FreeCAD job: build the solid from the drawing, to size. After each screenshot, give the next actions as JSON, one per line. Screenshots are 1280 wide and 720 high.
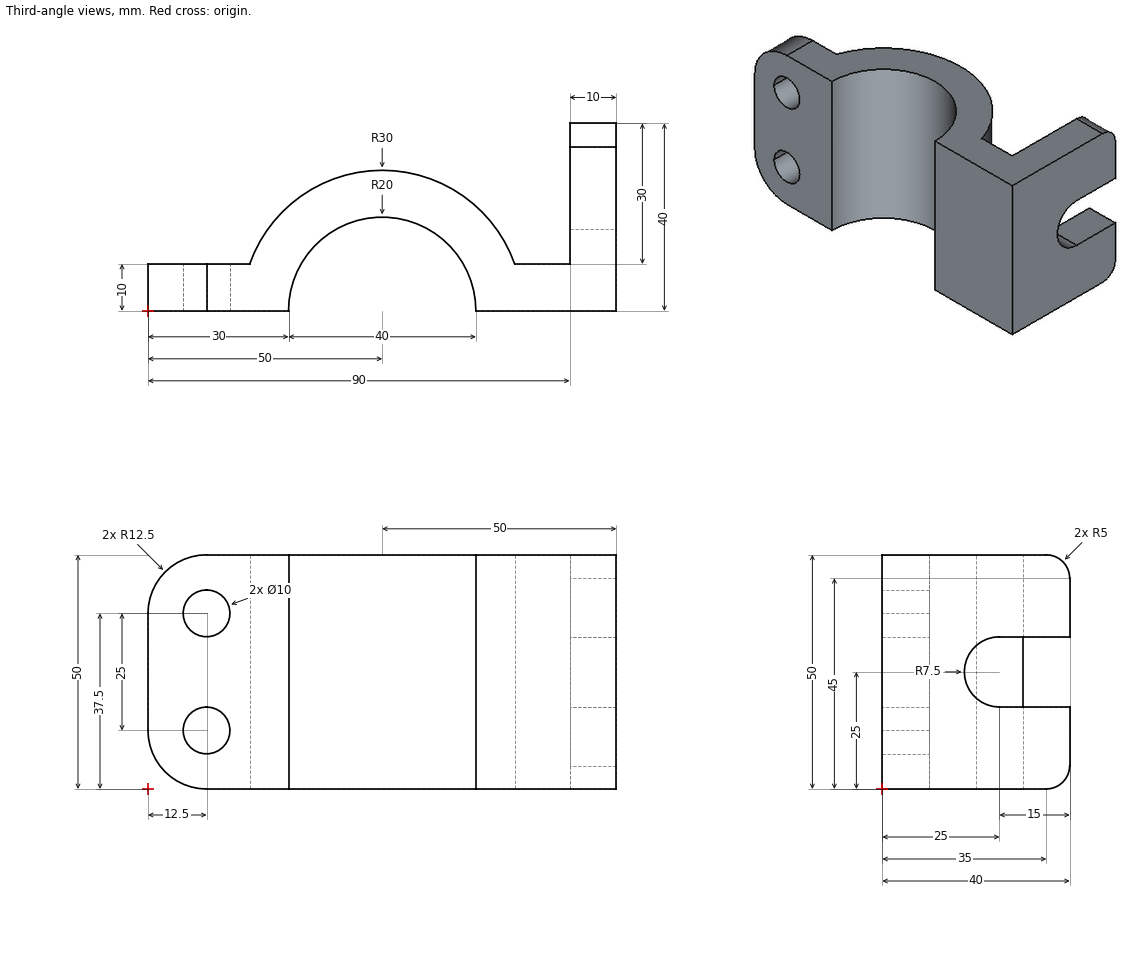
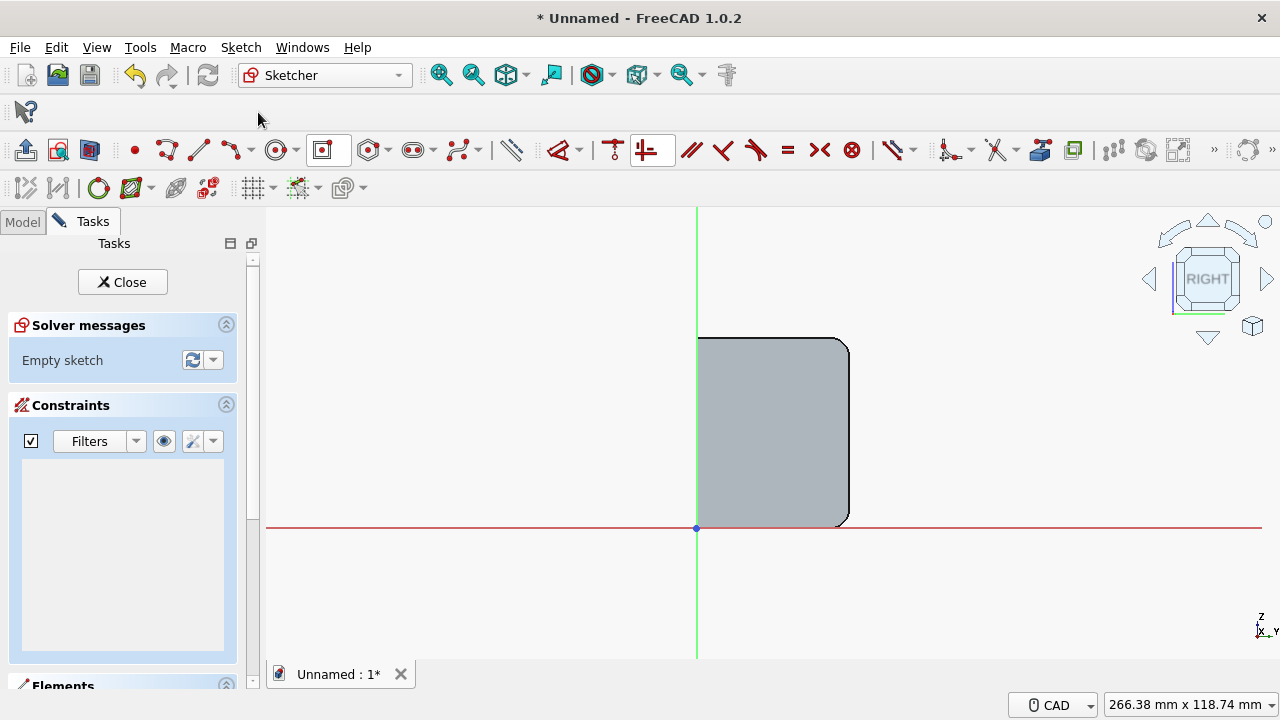
{"action": "scroll", "coordinate": [829, 493], "scroll_direction": "up", "scroll_amount": 4}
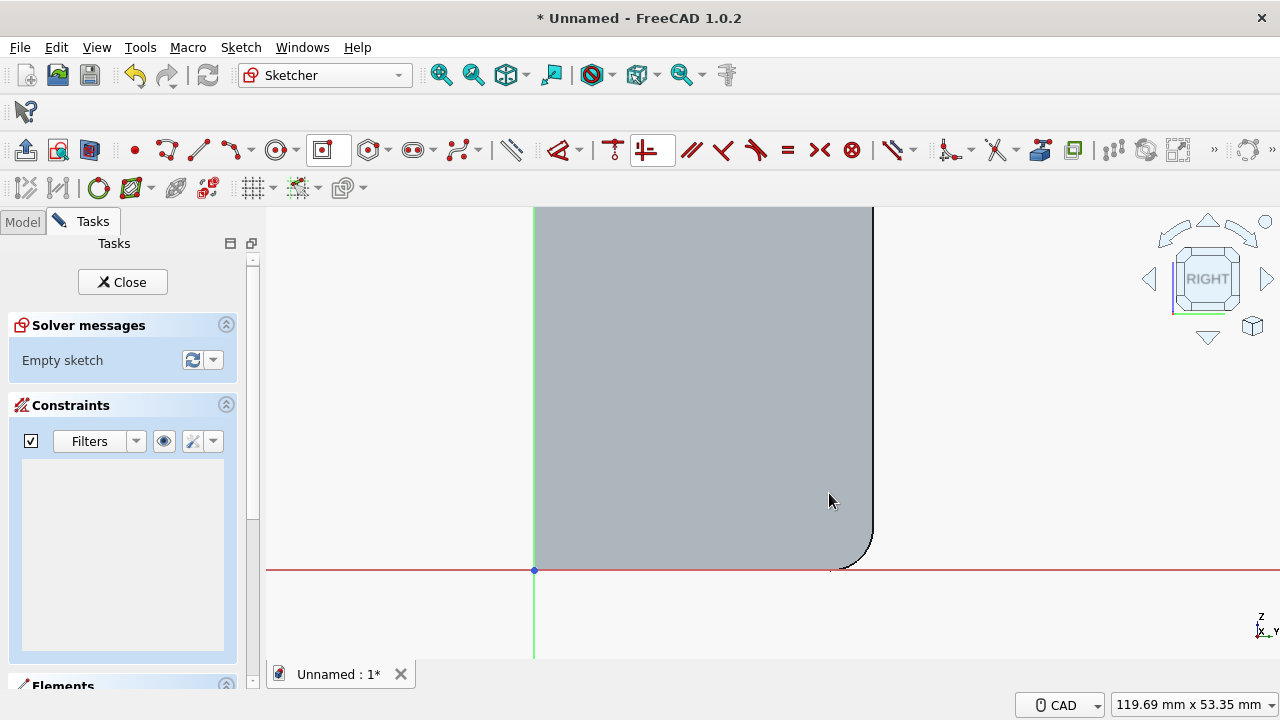
{"action": "left_click", "coordinate": [168, 150]}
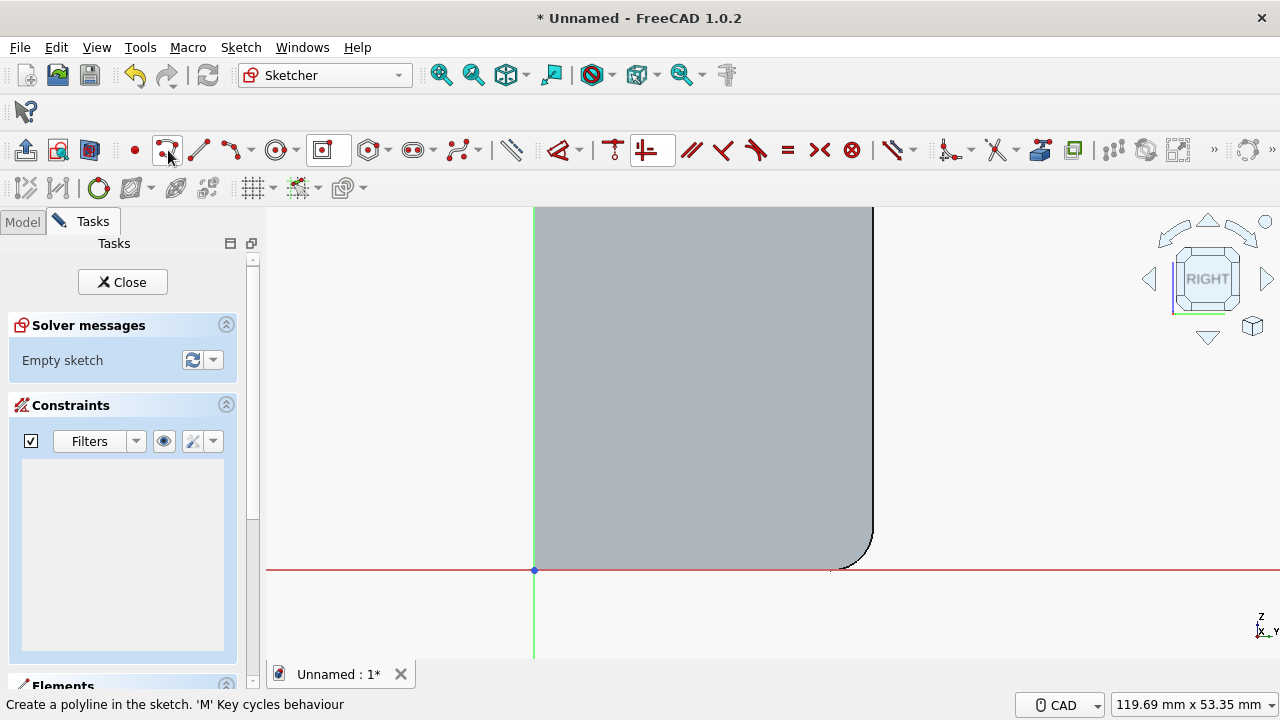
{"action": "left_click", "coordinate": [746, 422]}
{"action": "left_click", "coordinate": [873, 422]}
{"action": "left_click", "coordinate": [873, 295]}
{"action": "left_click", "coordinate": [746, 295]}
{"action": "right_click", "coordinate": [746, 295]}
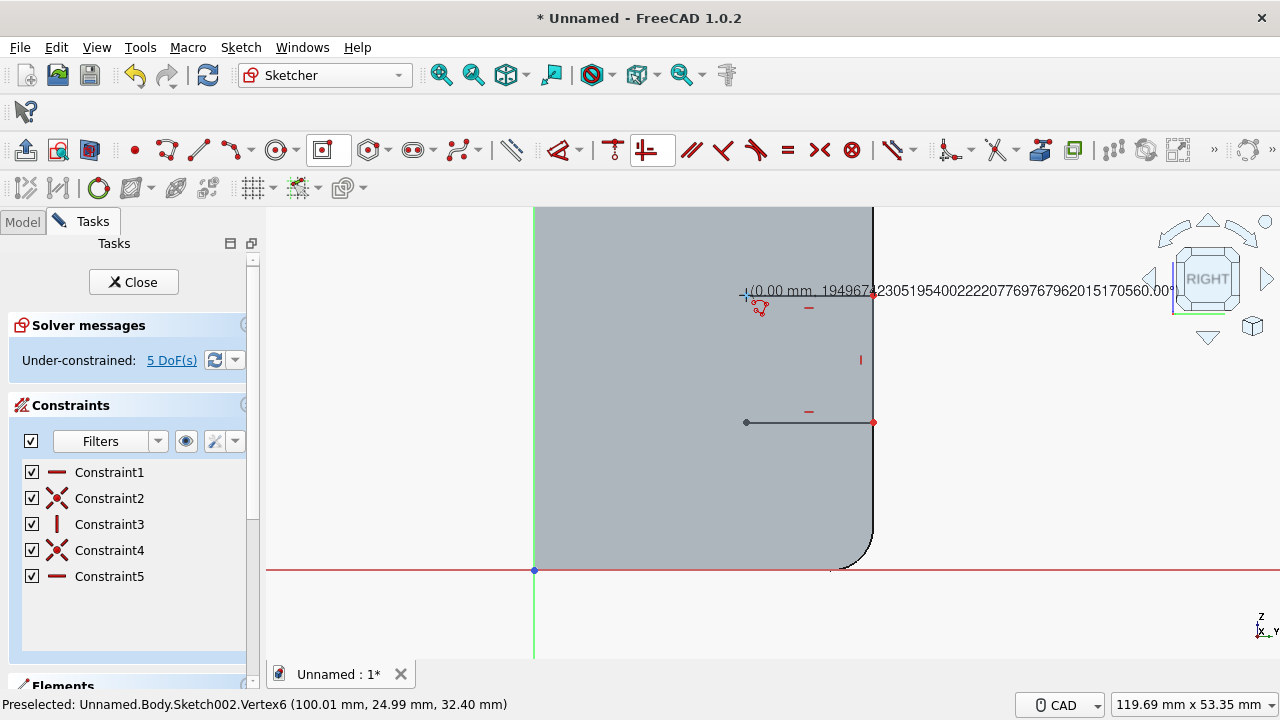
{"action": "left_click", "coordinate": [232, 150]}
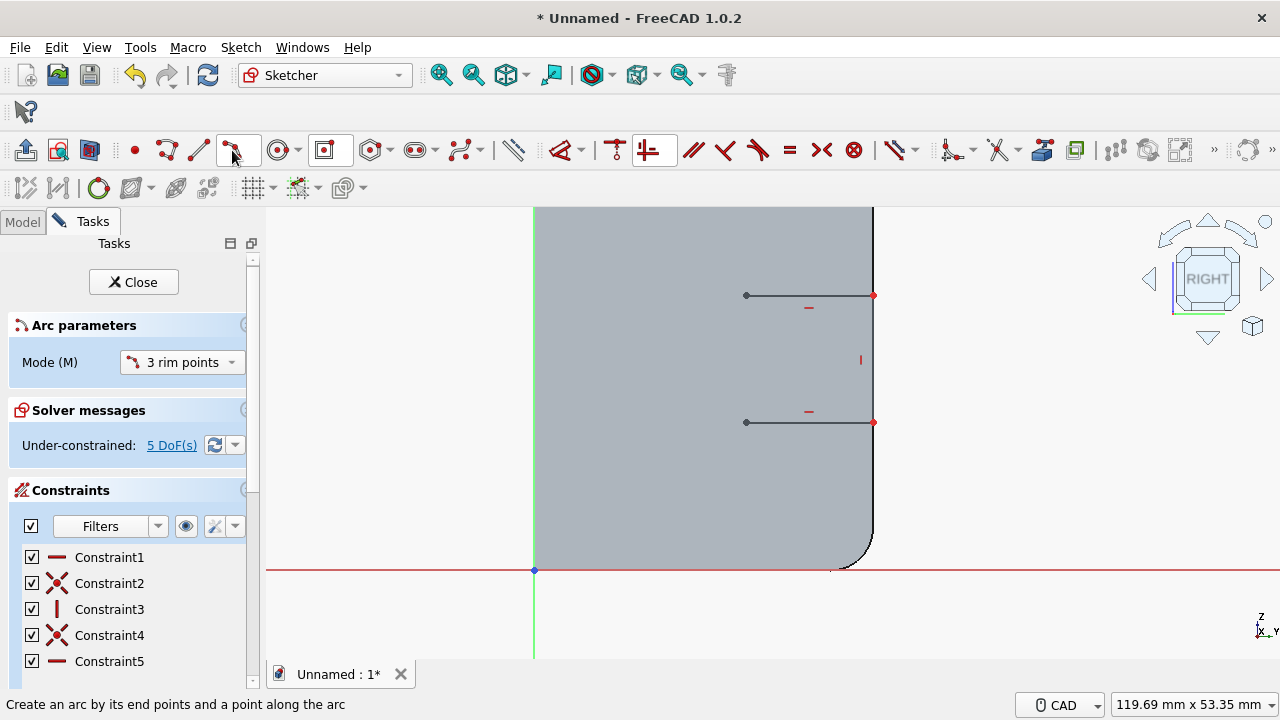
{"action": "left_click", "coordinate": [746, 296]}
{"action": "left_click", "coordinate": [746, 423]}
{"action": "left_click", "coordinate": [683, 359]}
{"action": "key", "text": "Escape"}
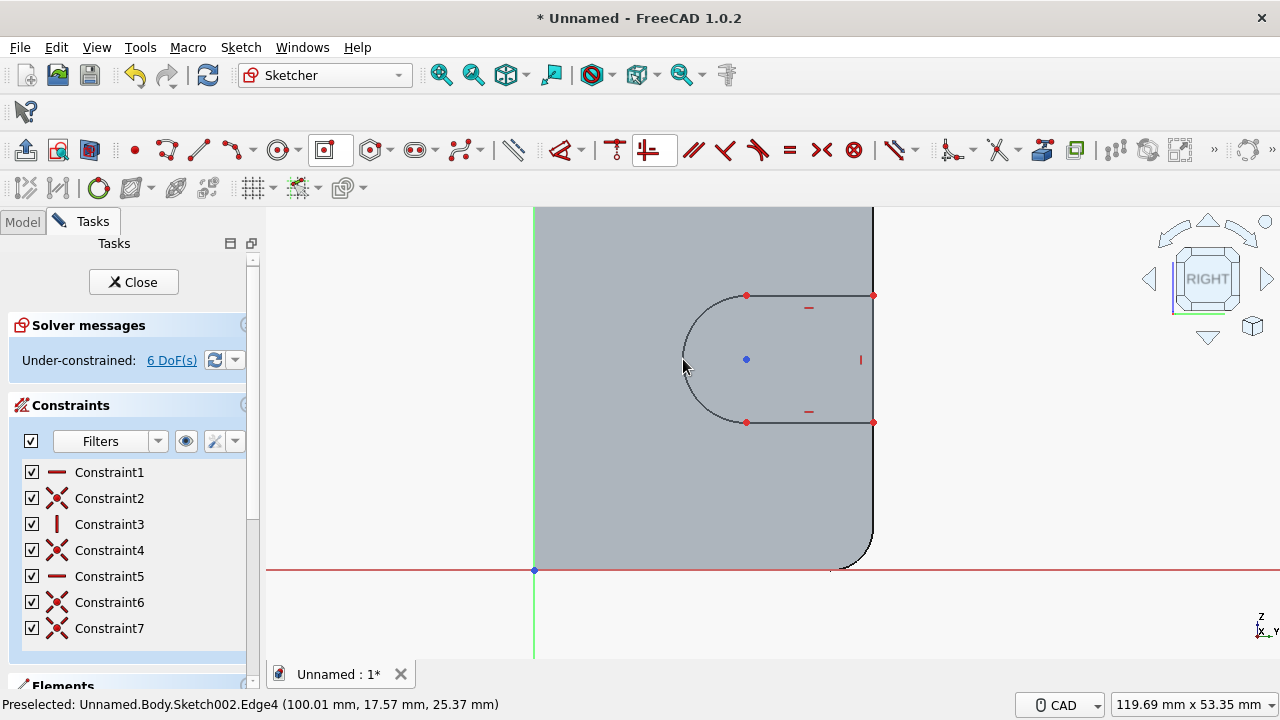
{"action": "left_click", "coordinate": [784, 423]}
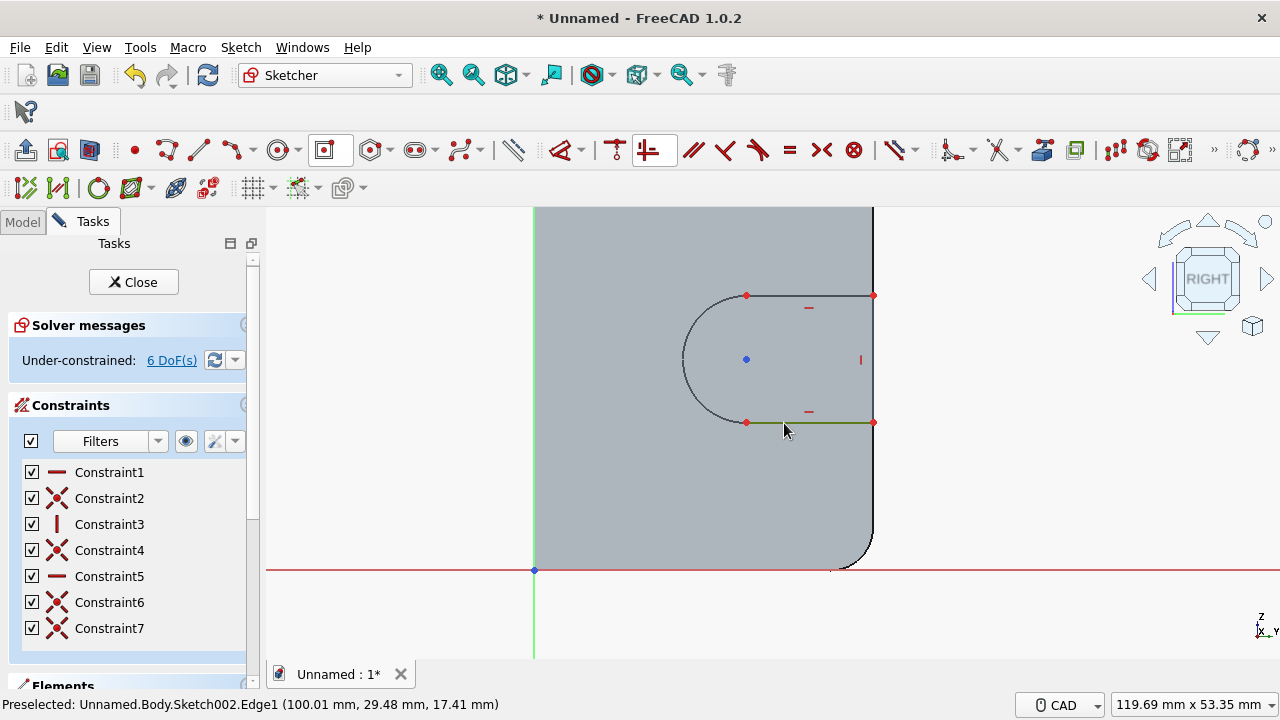
{"action": "left_click", "coordinate": [695, 322]}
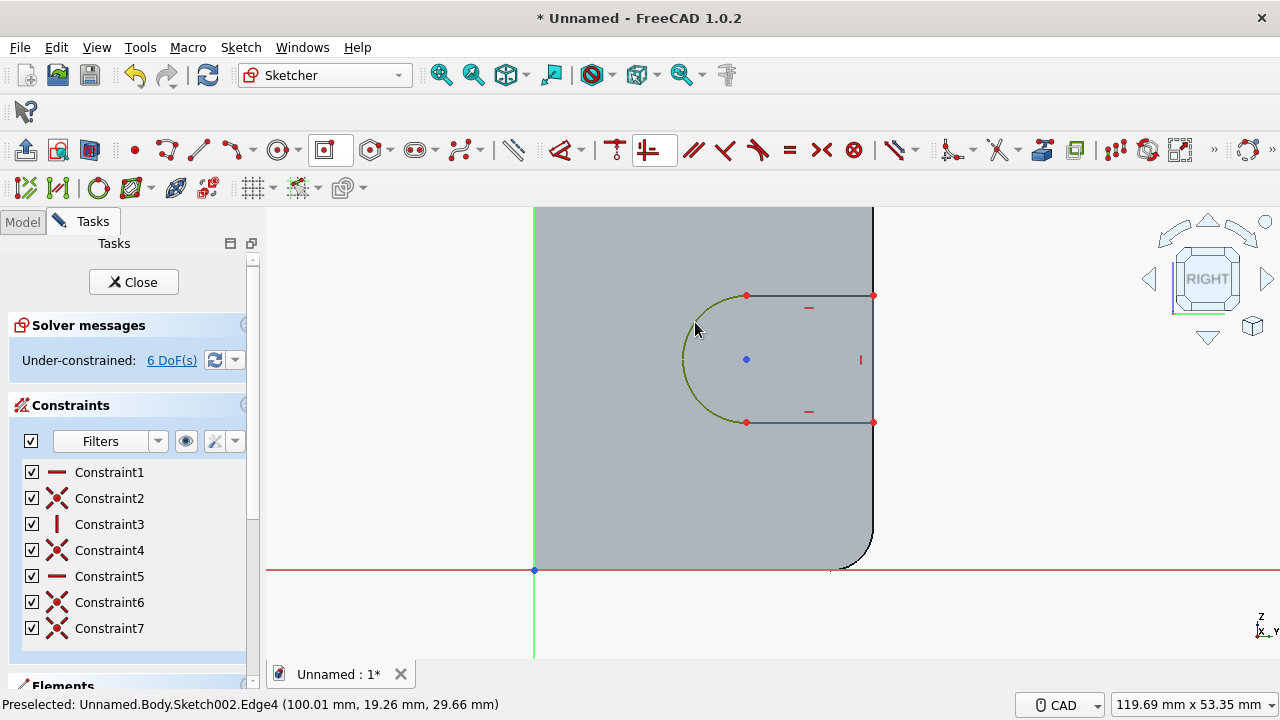
{"action": "left_click", "coordinate": [758, 150]}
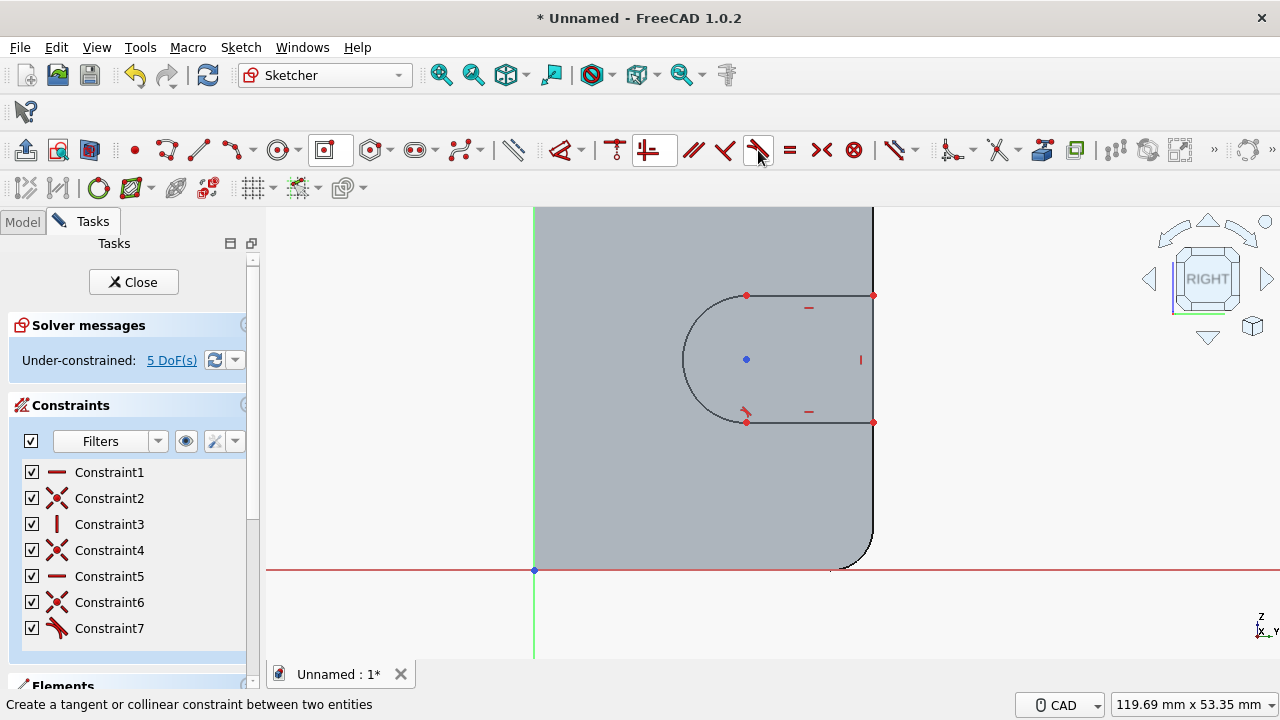
{"action": "left_click", "coordinate": [835, 296]}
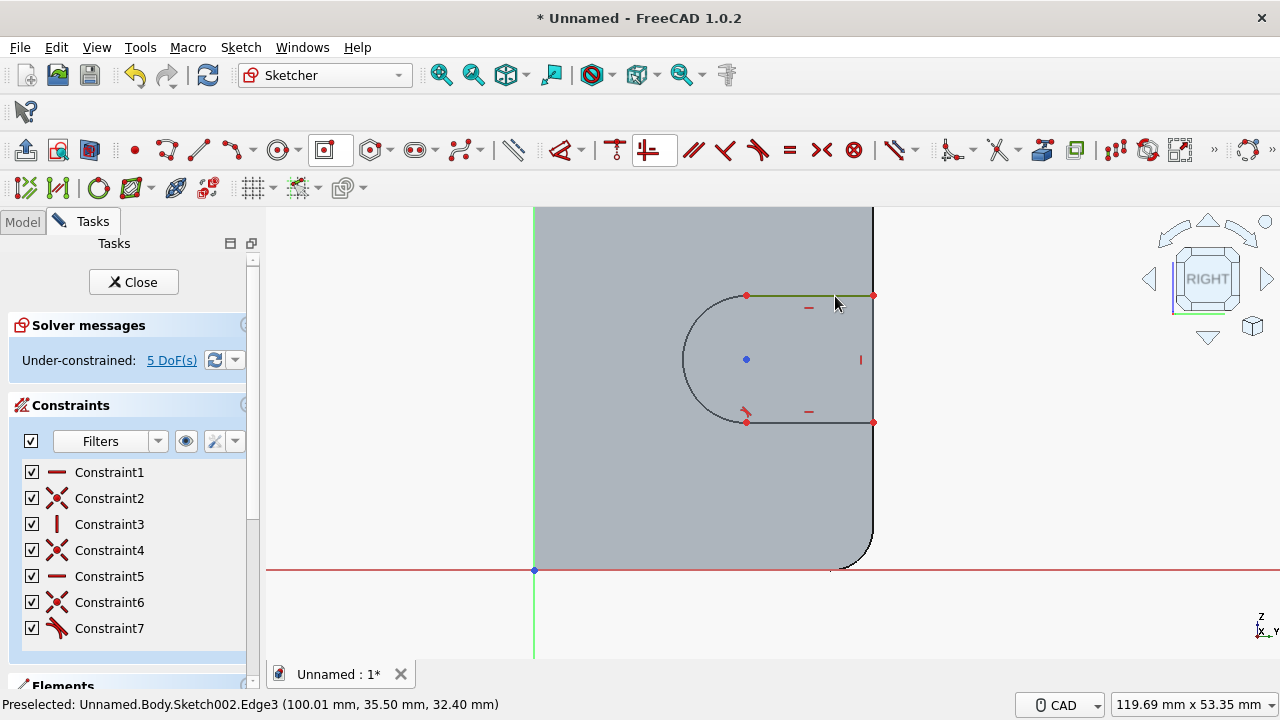
{"action": "left_click", "coordinate": [695, 322]}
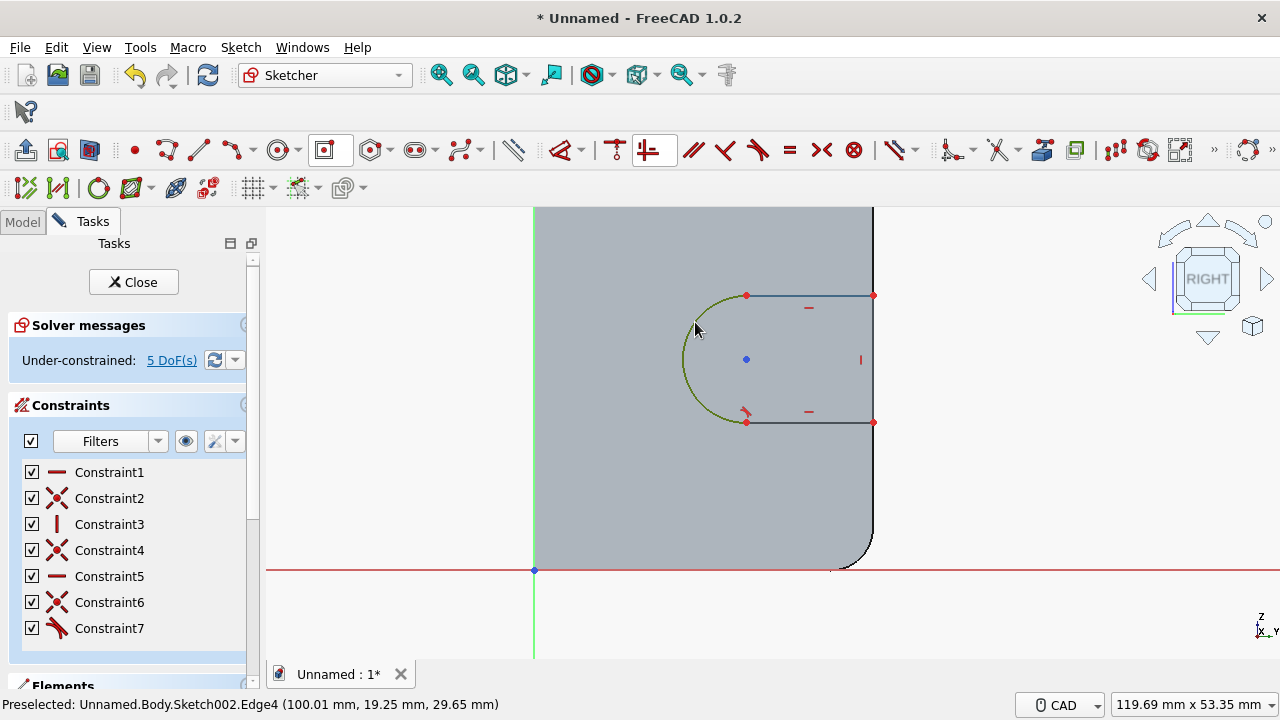
{"action": "left_click", "coordinate": [758, 150]}